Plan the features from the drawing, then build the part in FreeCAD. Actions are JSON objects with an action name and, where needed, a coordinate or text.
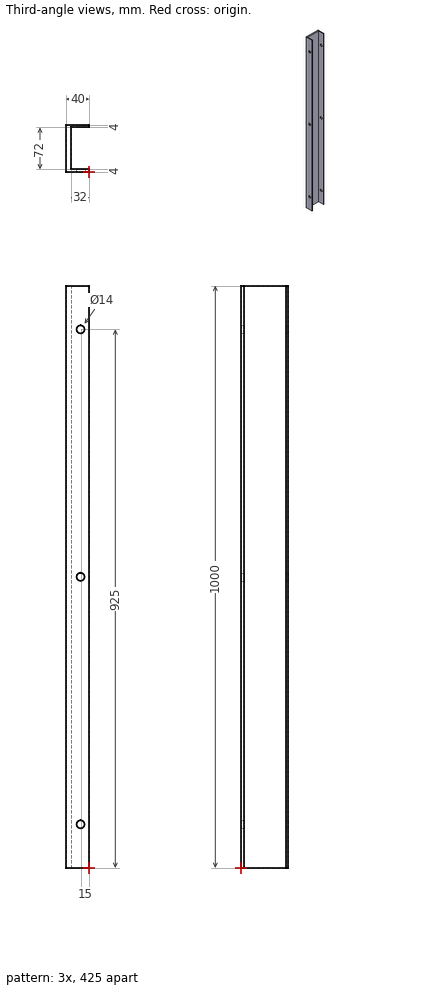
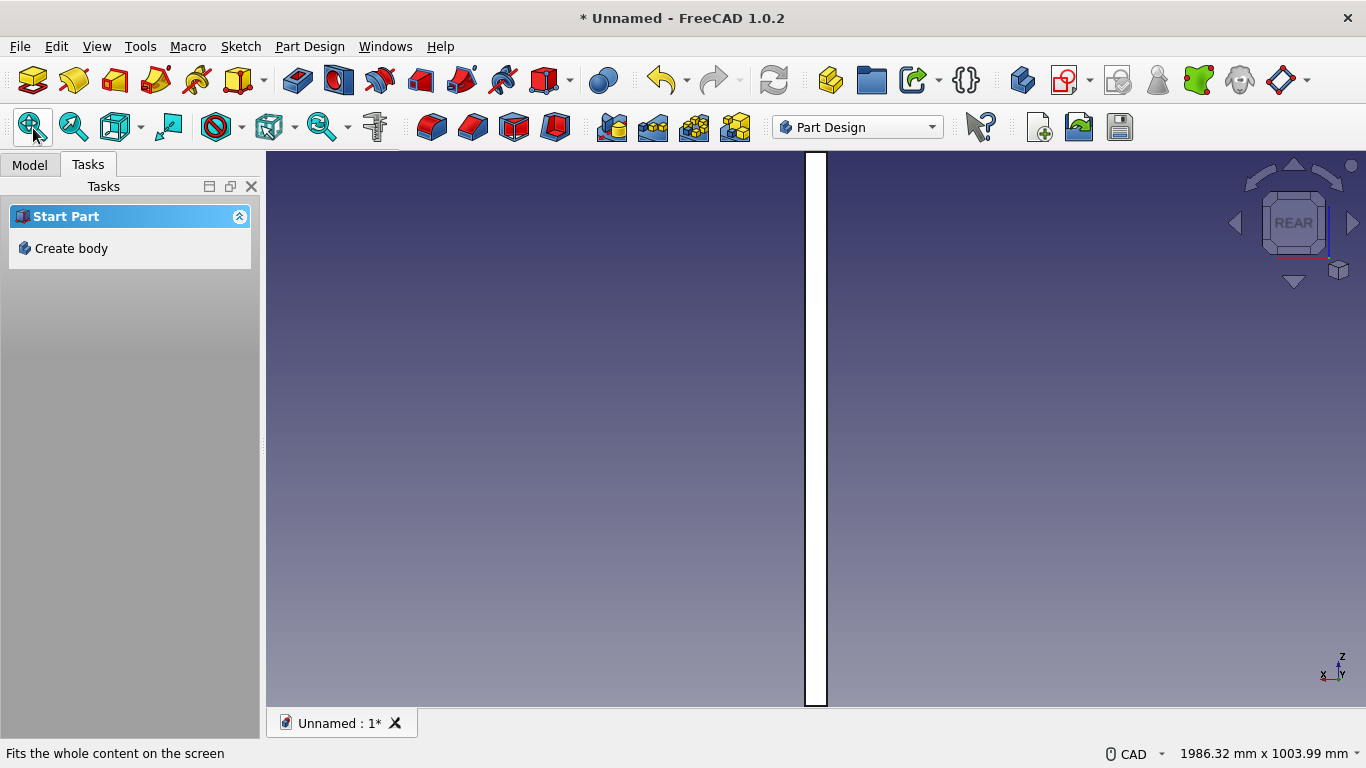
{"action": "left_click", "coordinate": [816, 191]}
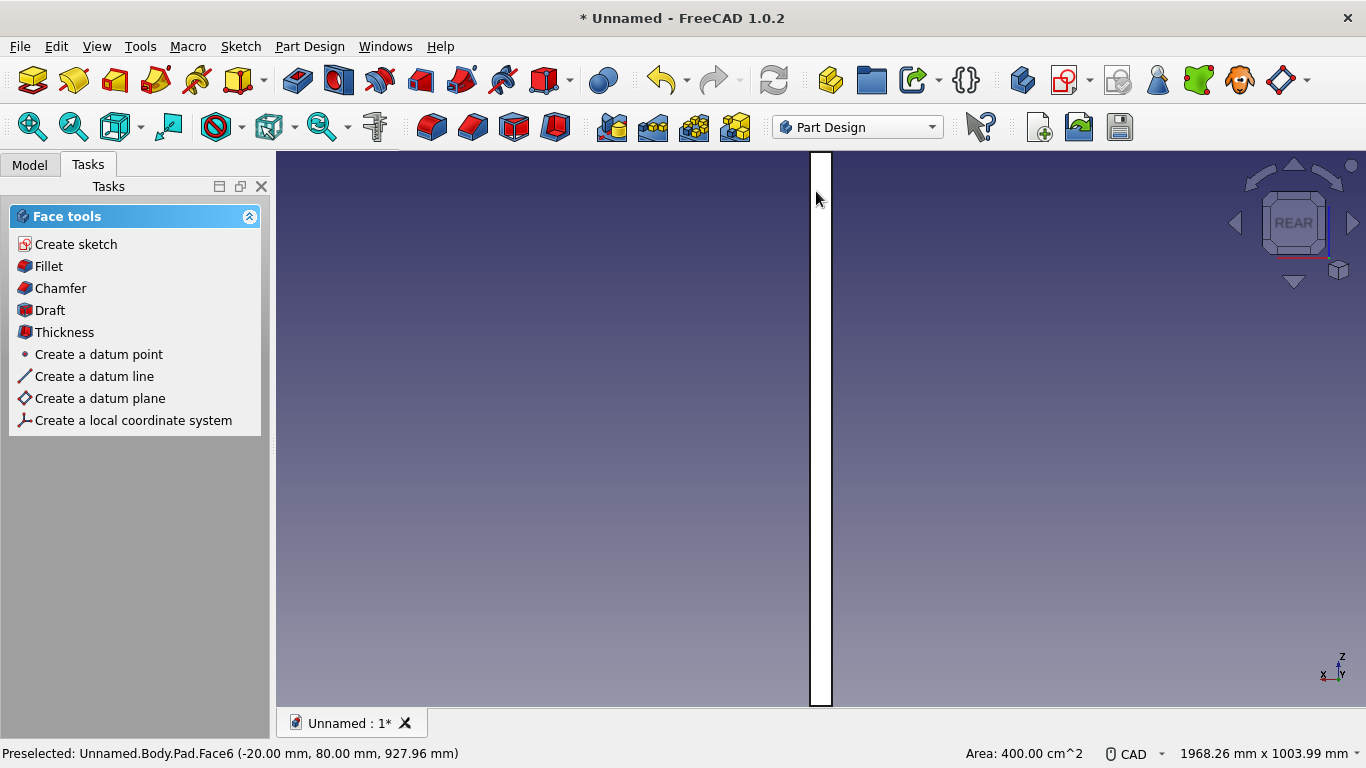
{"action": "left_click", "coordinate": [1064, 80]}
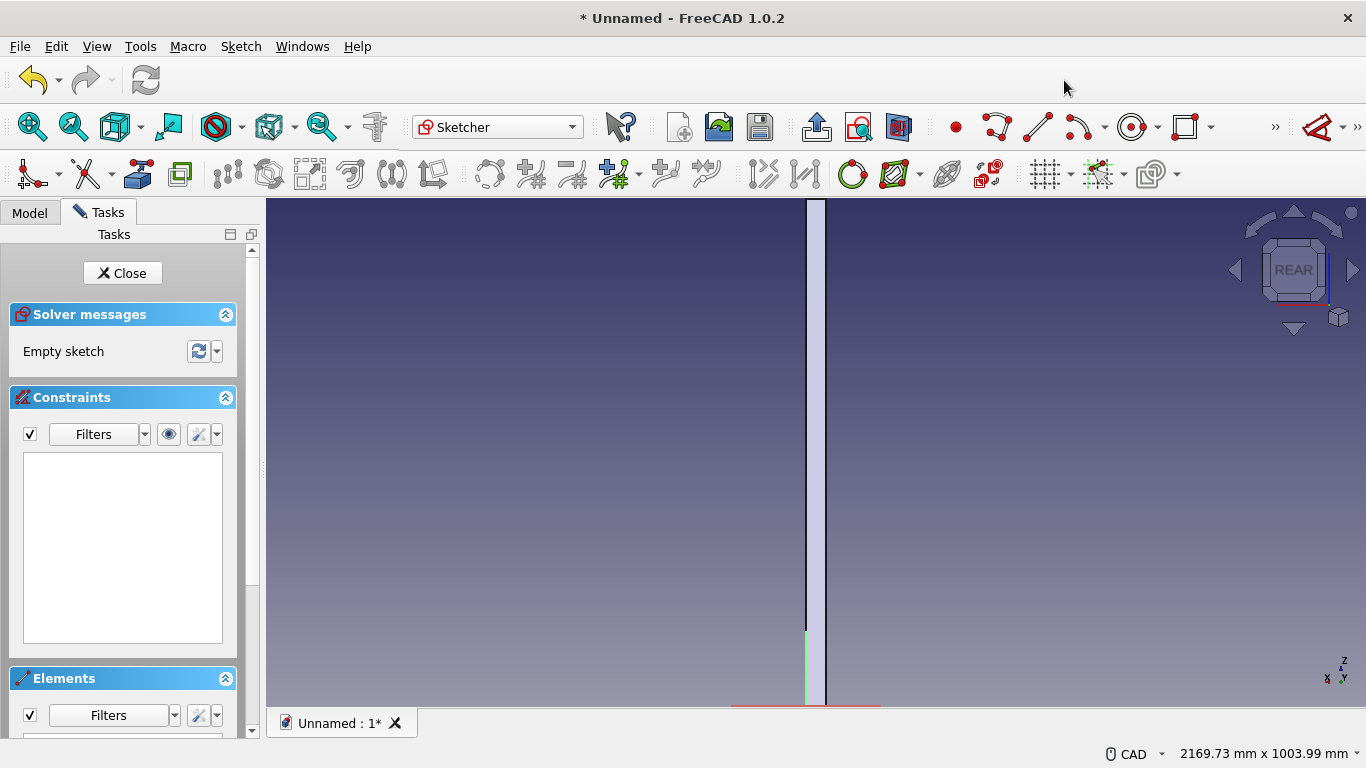
{"action": "scroll", "coordinate": [817, 226], "scroll_direction": "up", "scroll_amount": 15}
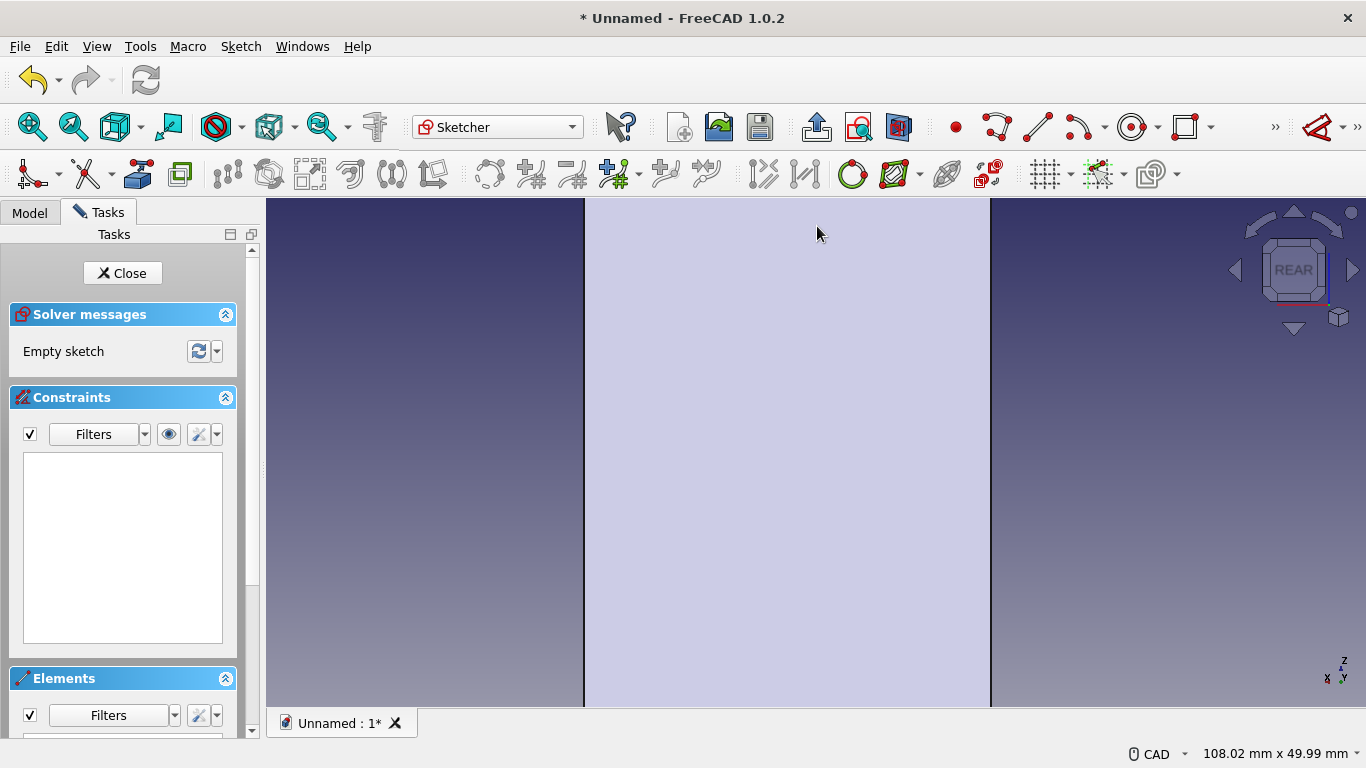
{"action": "scroll", "coordinate": [727, 442], "scroll_direction": "up", "scroll_amount": 4}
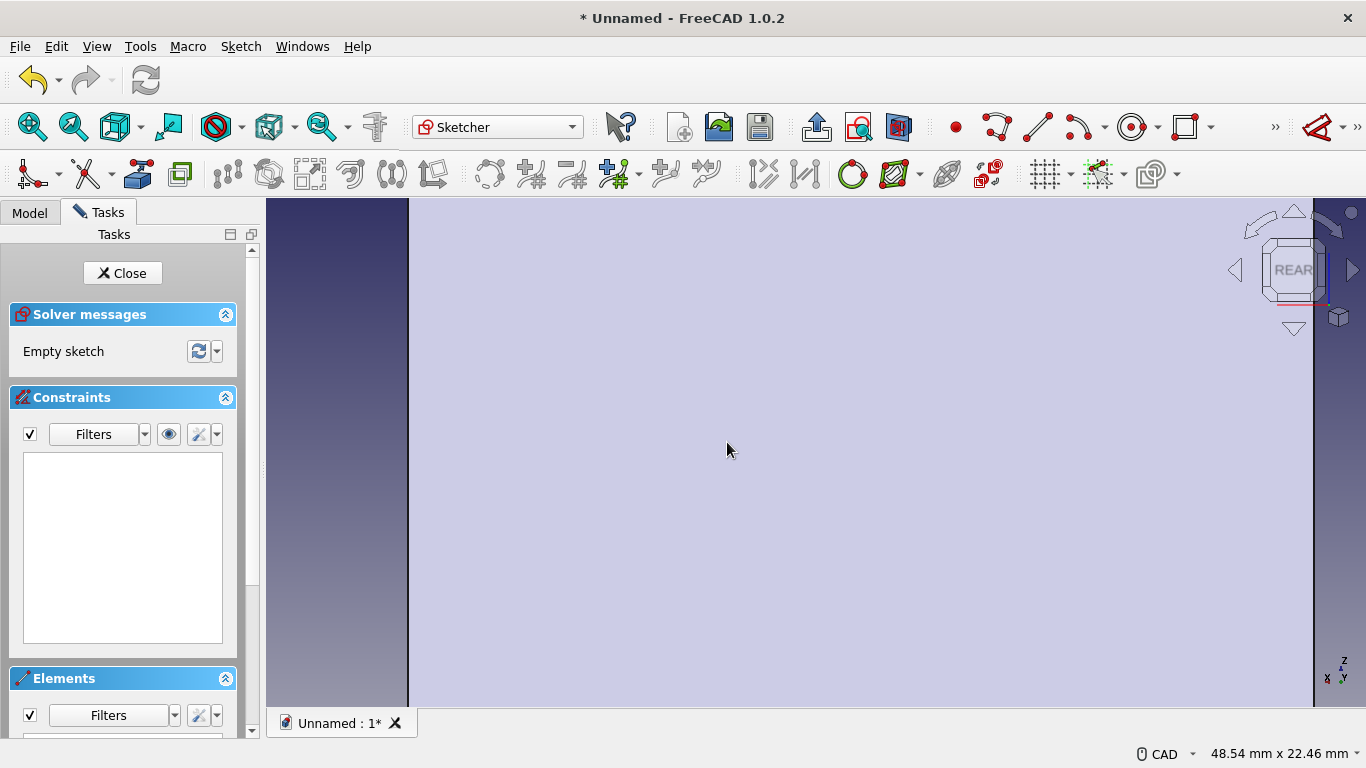
{"action": "left_click", "coordinate": [1132, 128]}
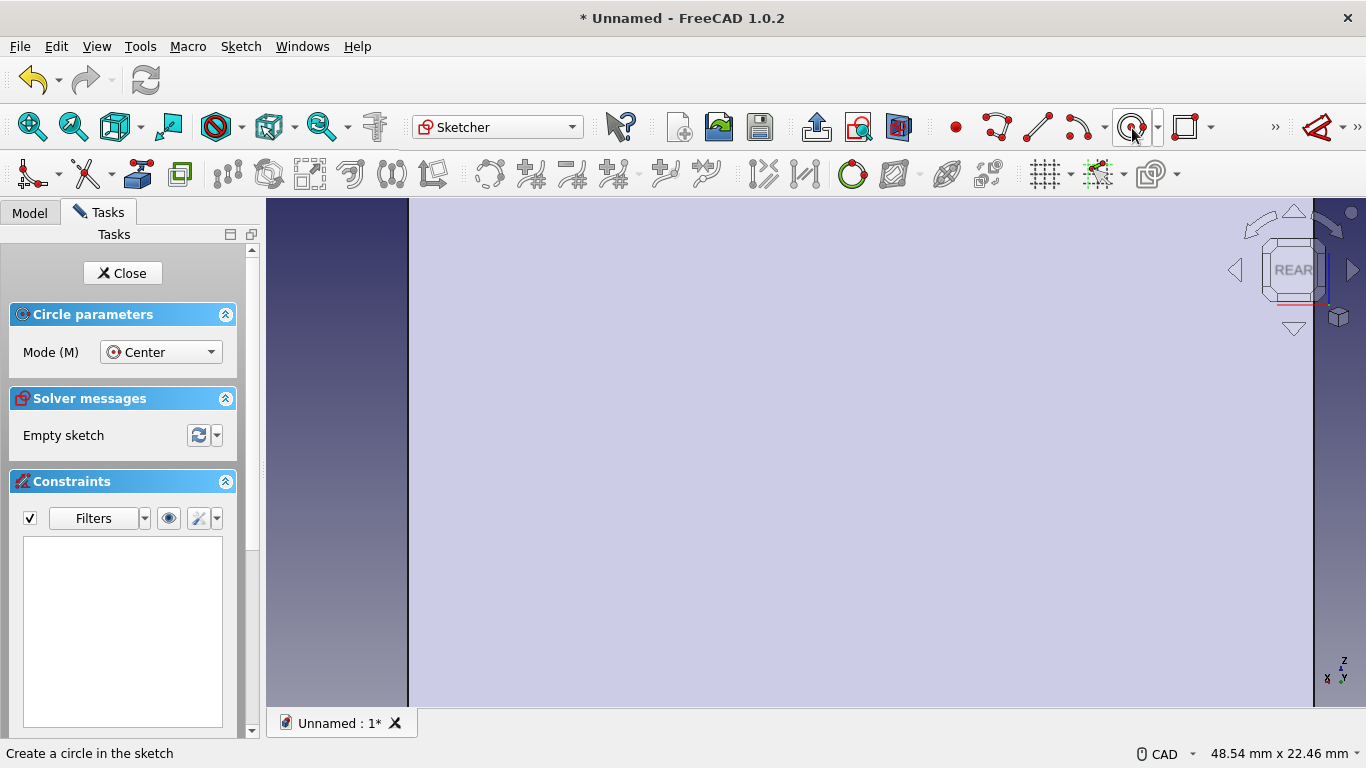
{"action": "left_click", "coordinate": [747, 452]}
{"action": "left_click", "coordinate": [860, 339]}
{"action": "key", "text": "Escape"}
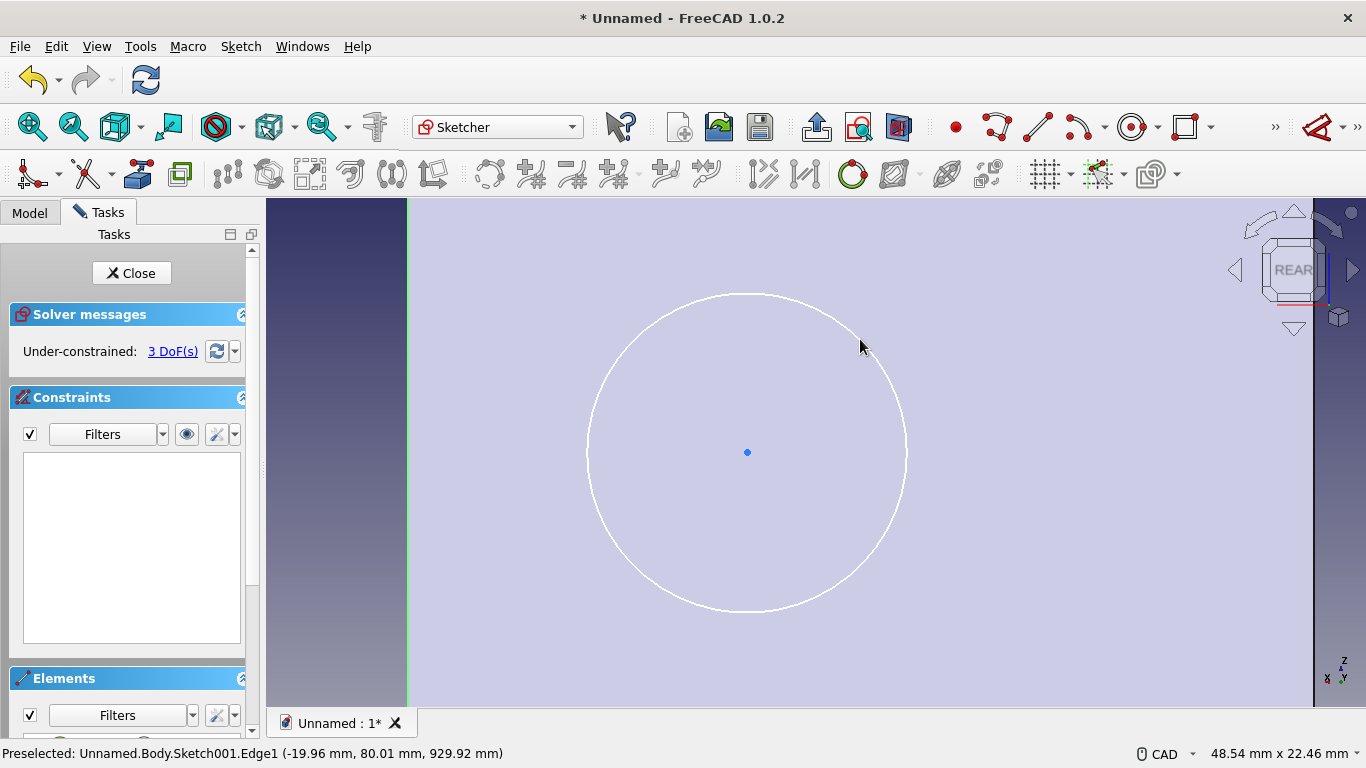
{"action": "left_click", "coordinate": [1316, 128]}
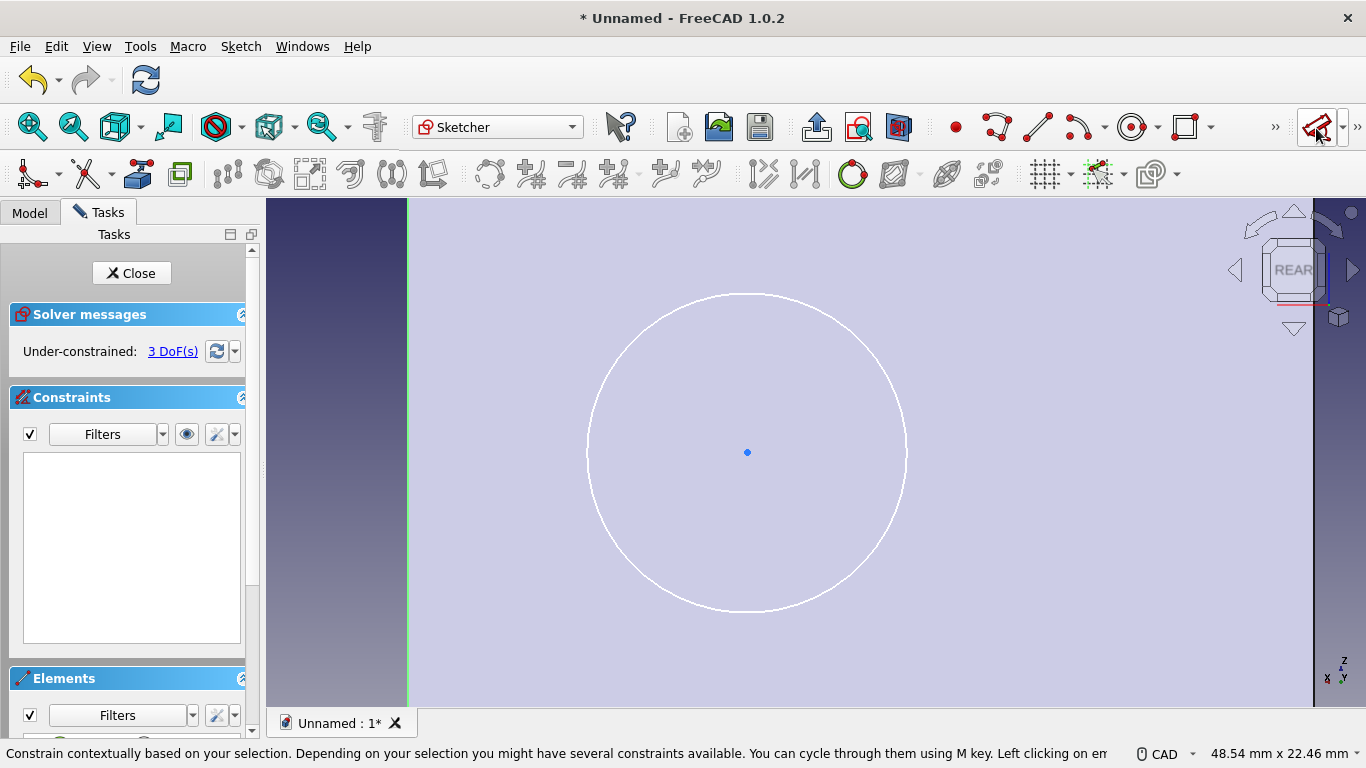
{"action": "left_click", "coordinate": [860, 340]}
{"action": "left_click", "coordinate": [883, 317]}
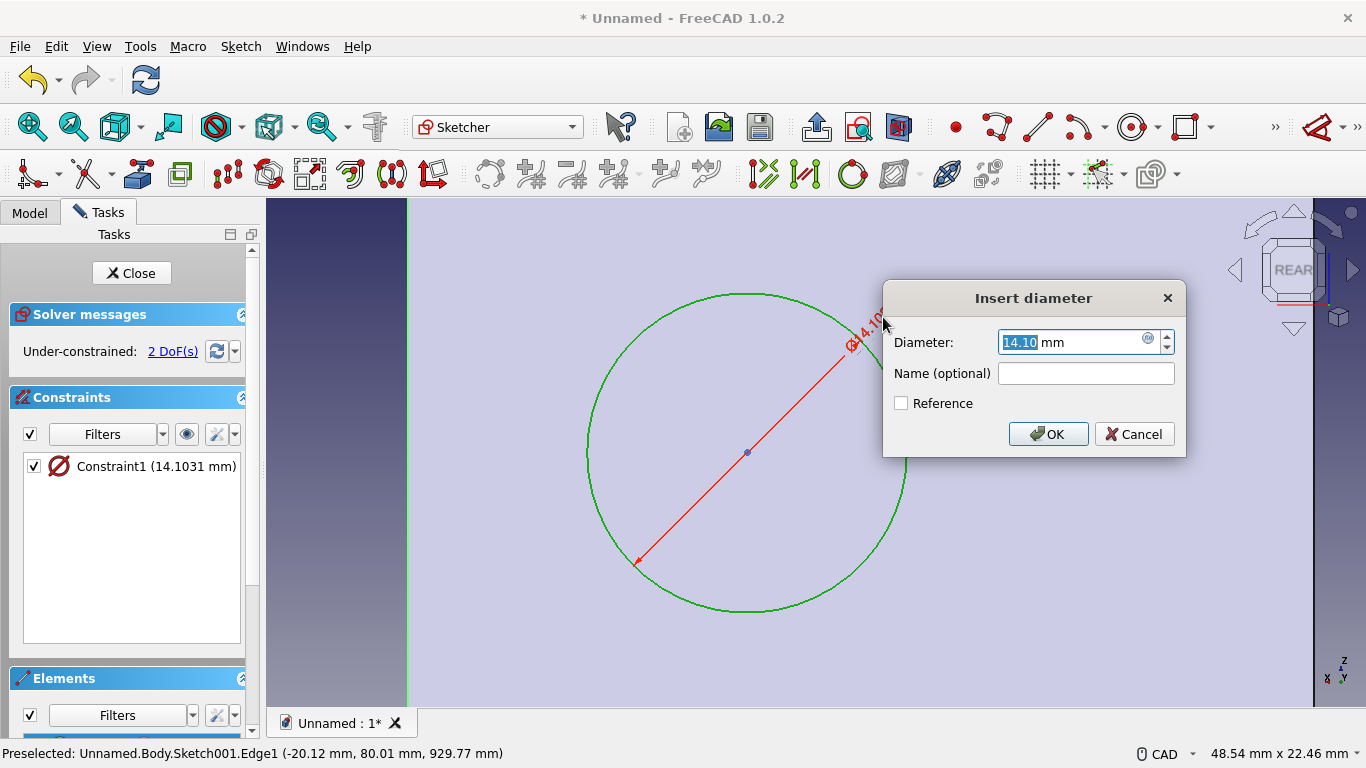
{"action": "type", "text": "14"}
{"action": "key", "text": "Return"}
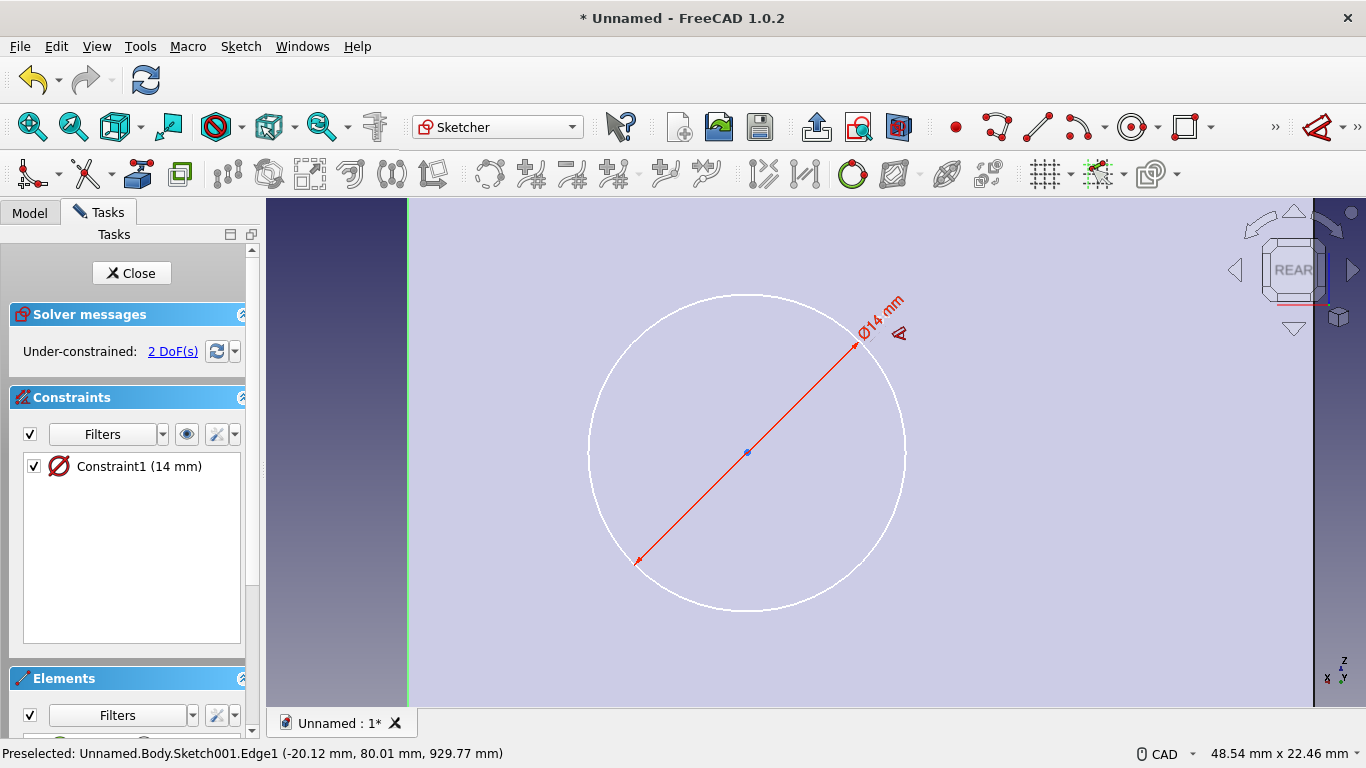
{"action": "left_click", "coordinate": [747, 453]}
{"action": "left_click", "coordinate": [577, 419]}